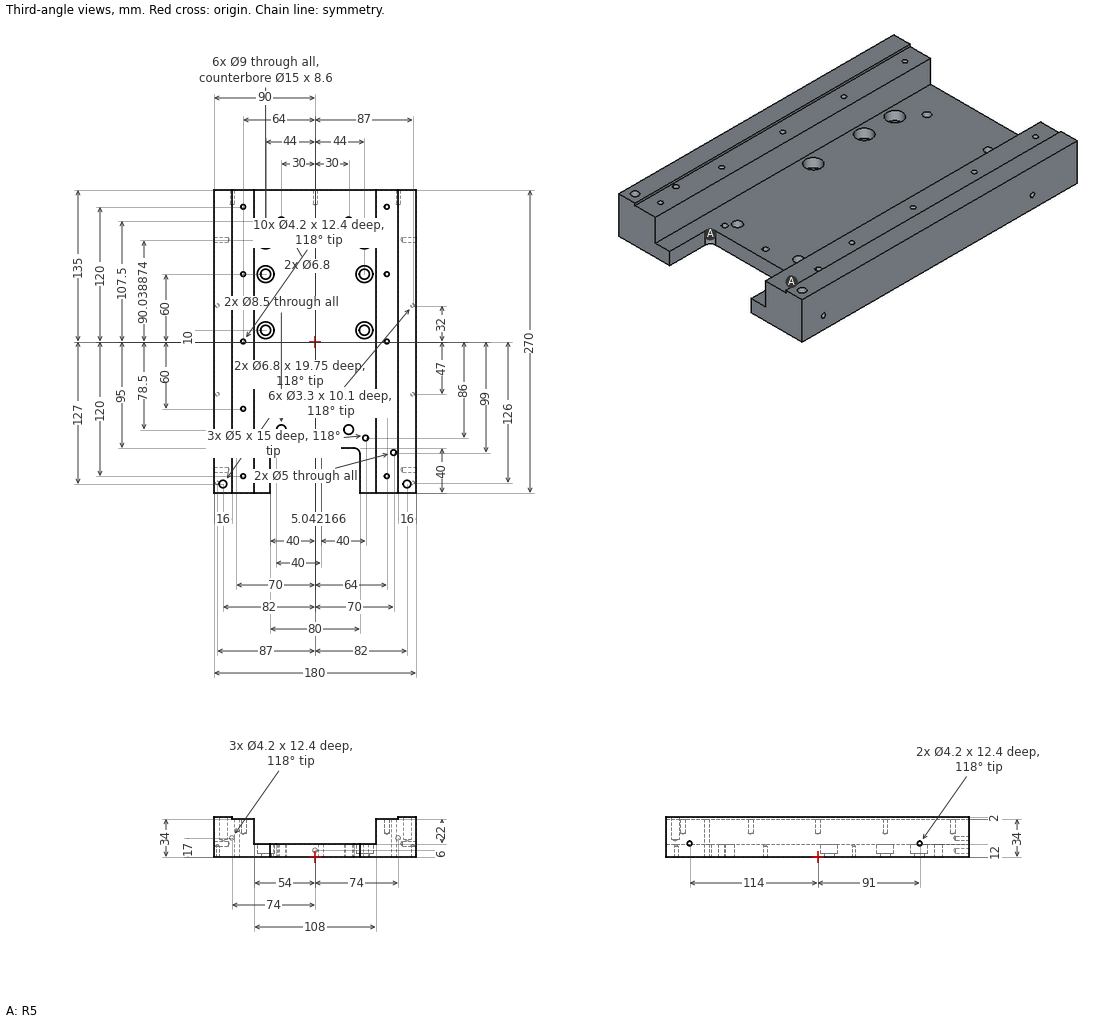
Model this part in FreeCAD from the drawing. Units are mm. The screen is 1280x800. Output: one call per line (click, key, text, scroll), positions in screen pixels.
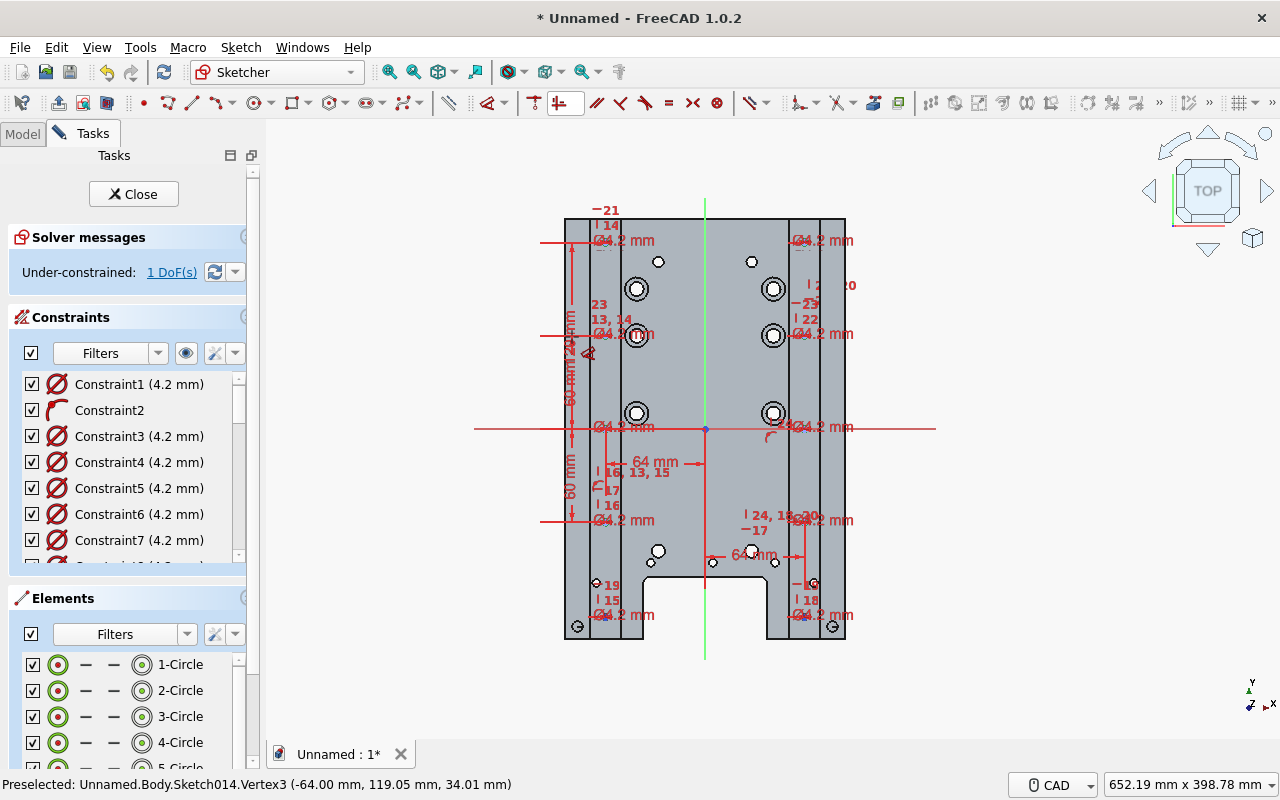
click(606, 617)
click(572, 523)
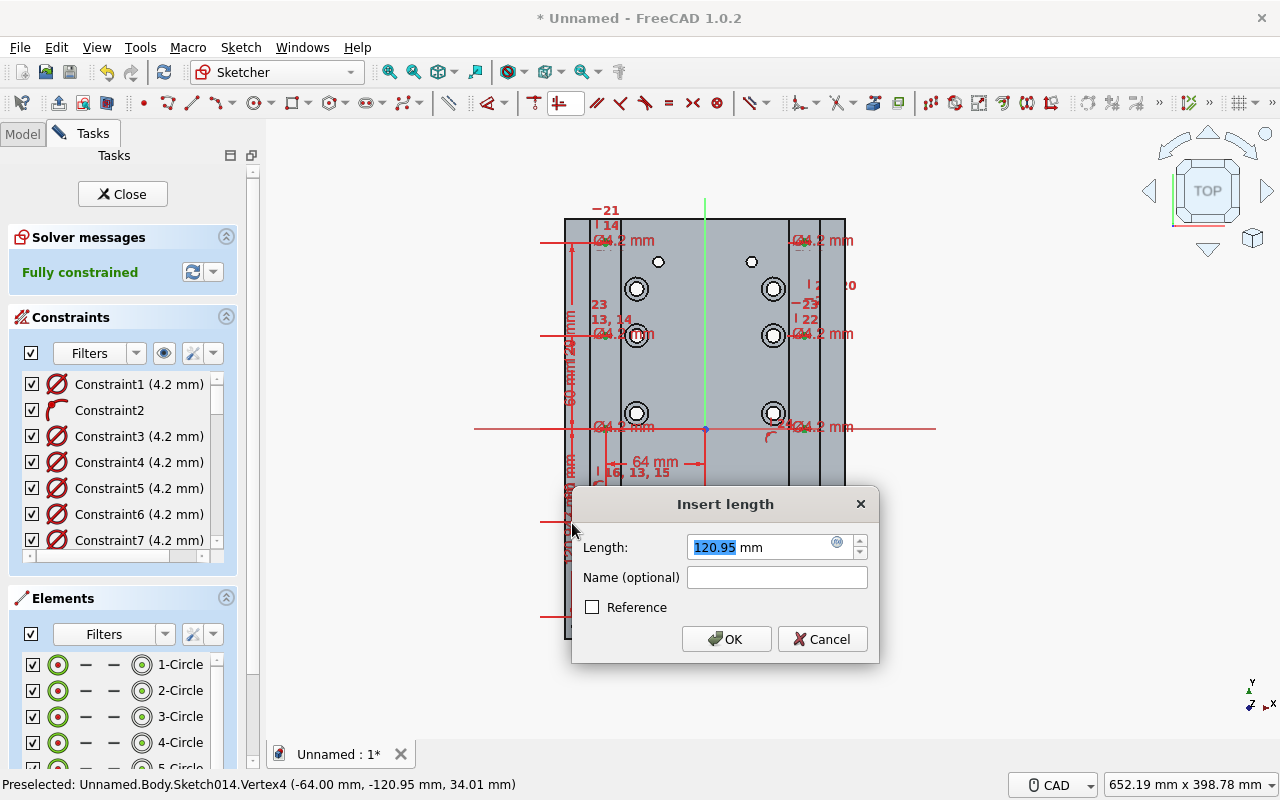
text(120)
key(Return)
key(Escape)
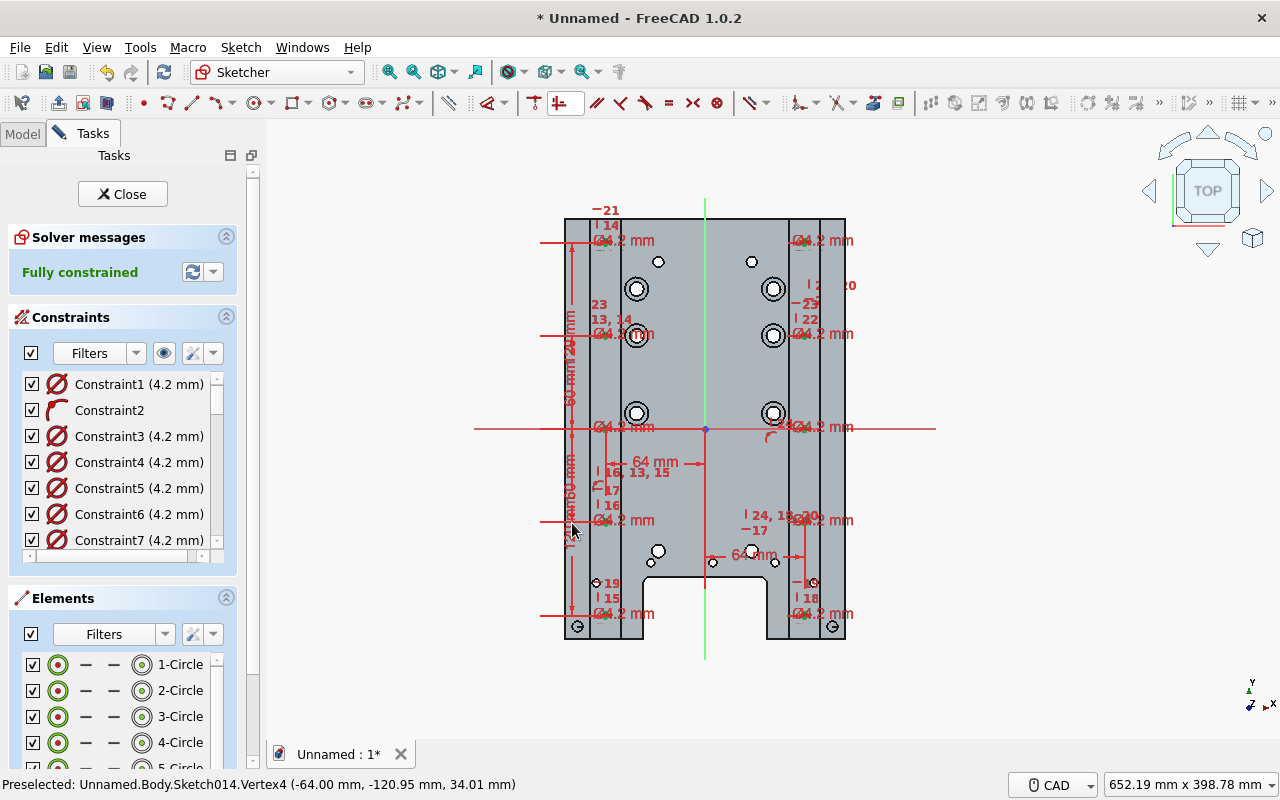
click(123, 194)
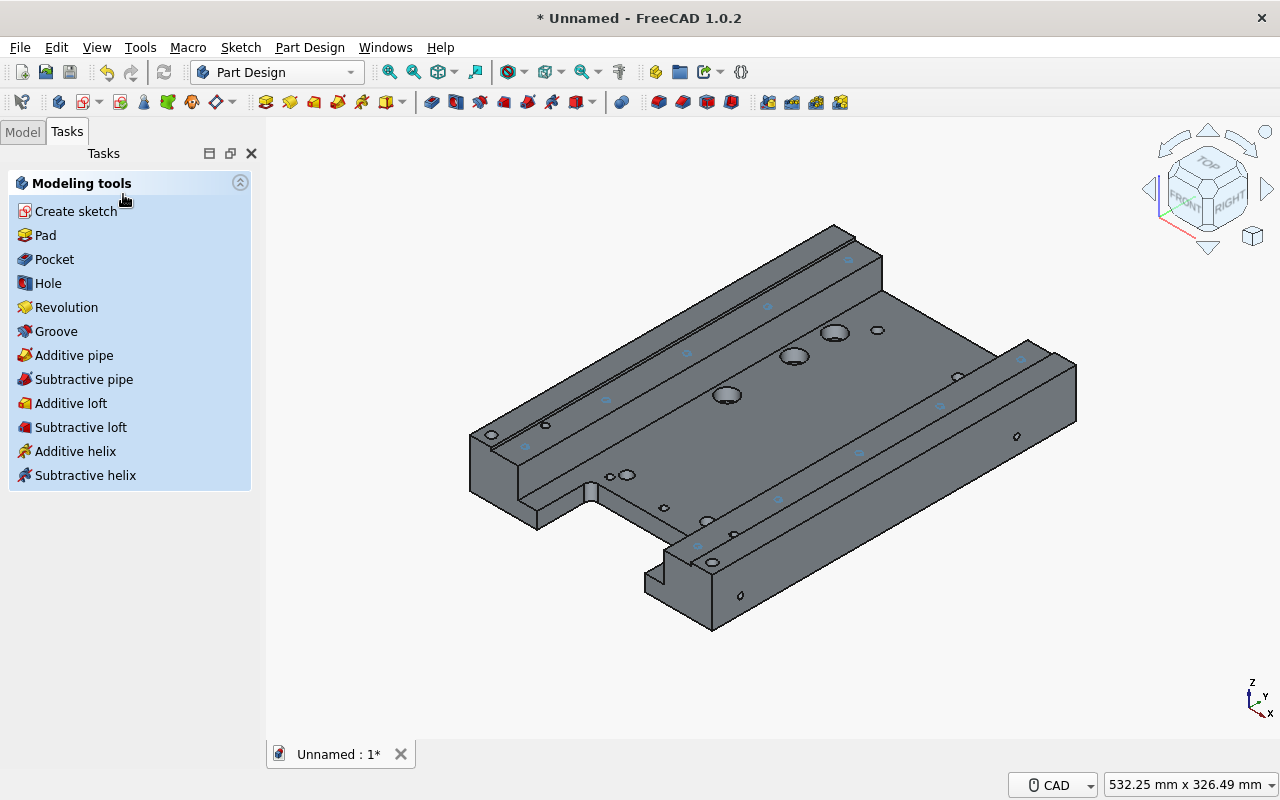
click(456, 102)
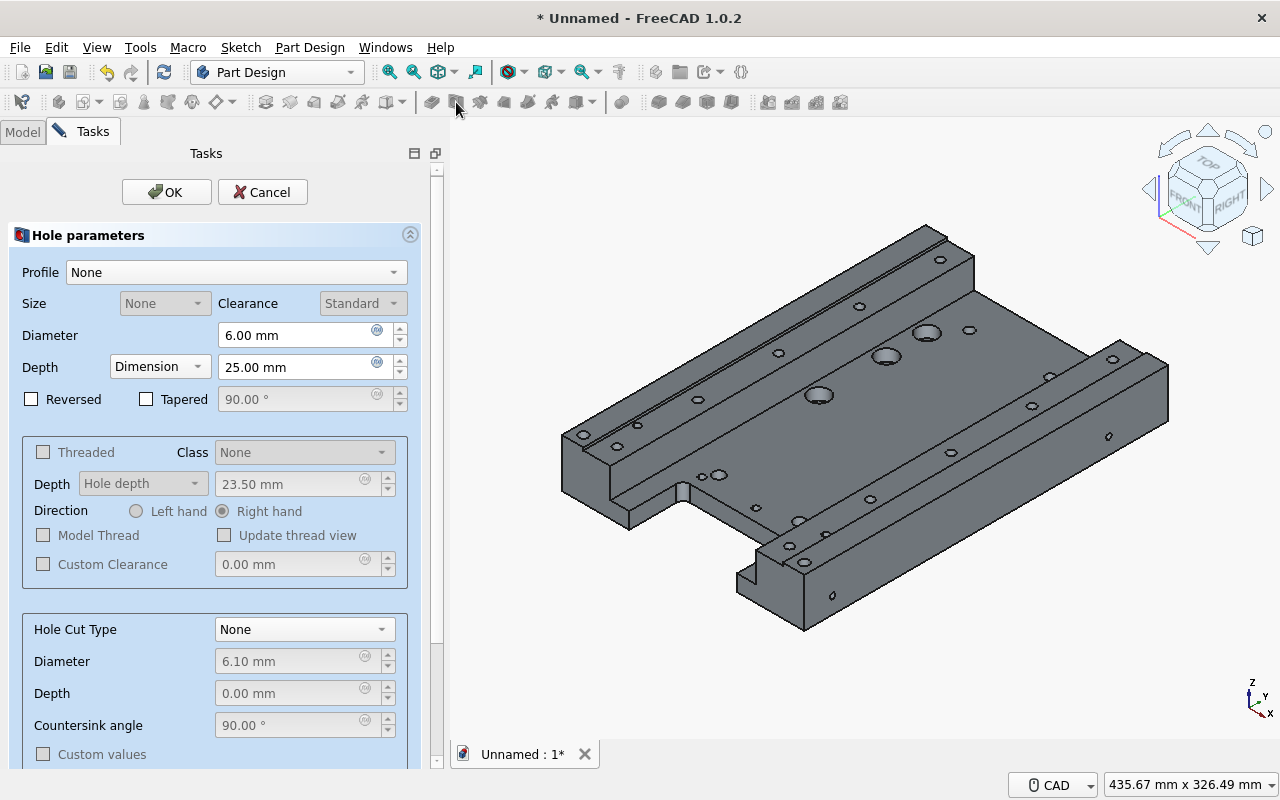
triple_click(305, 335)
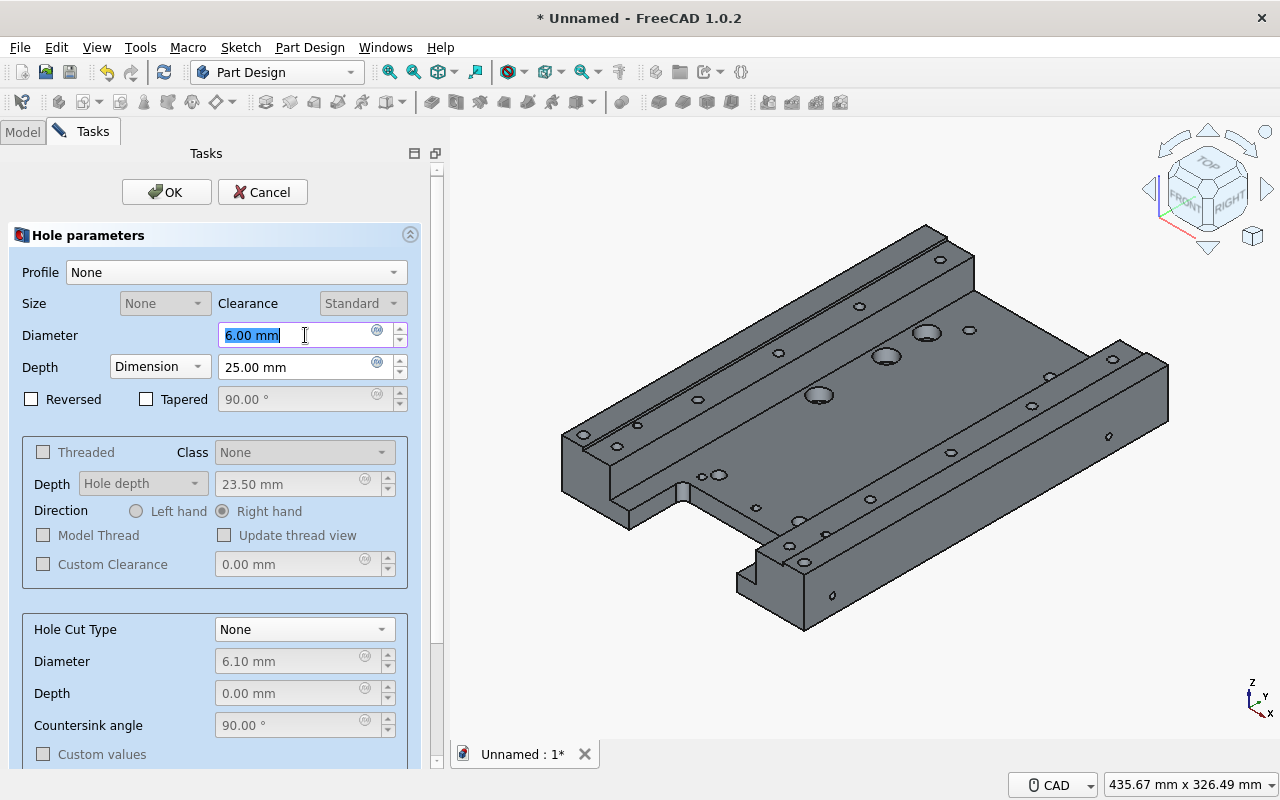
text(4.2)
key(Tab)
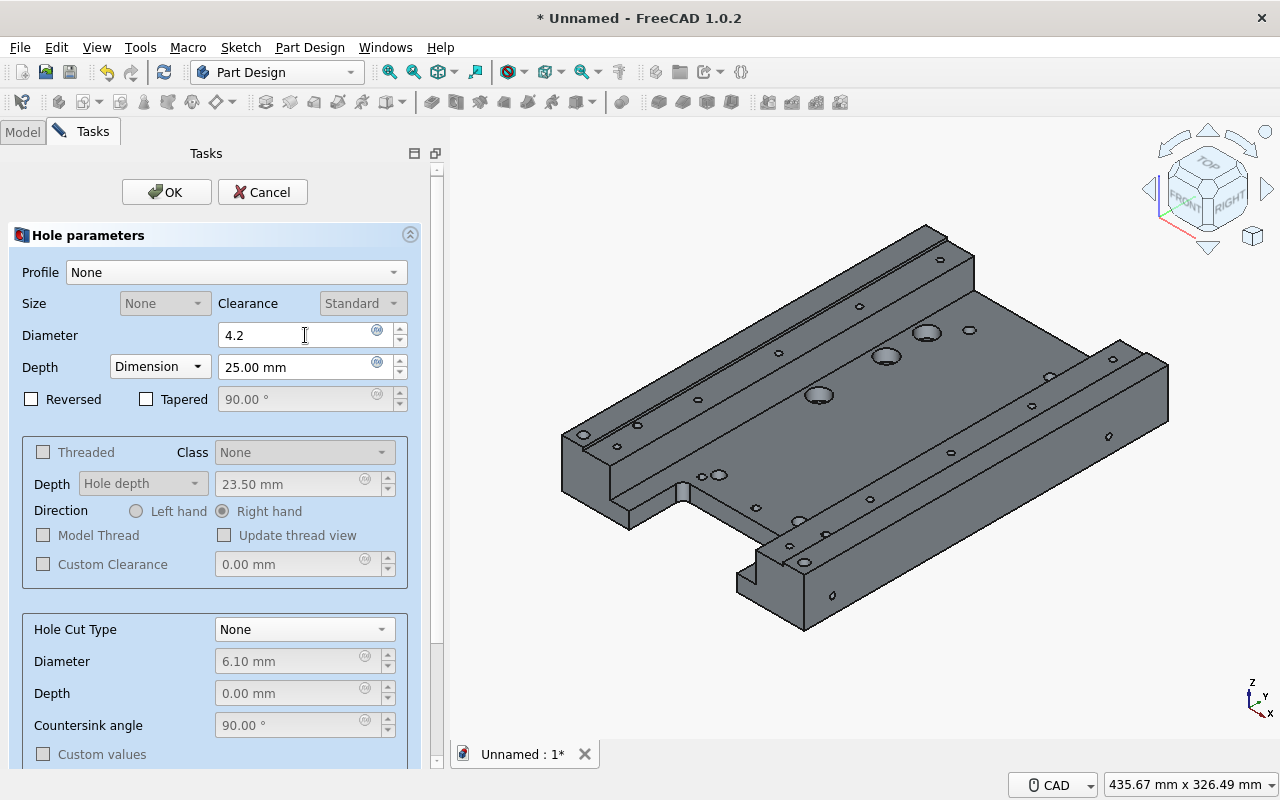
triple_click(305, 367)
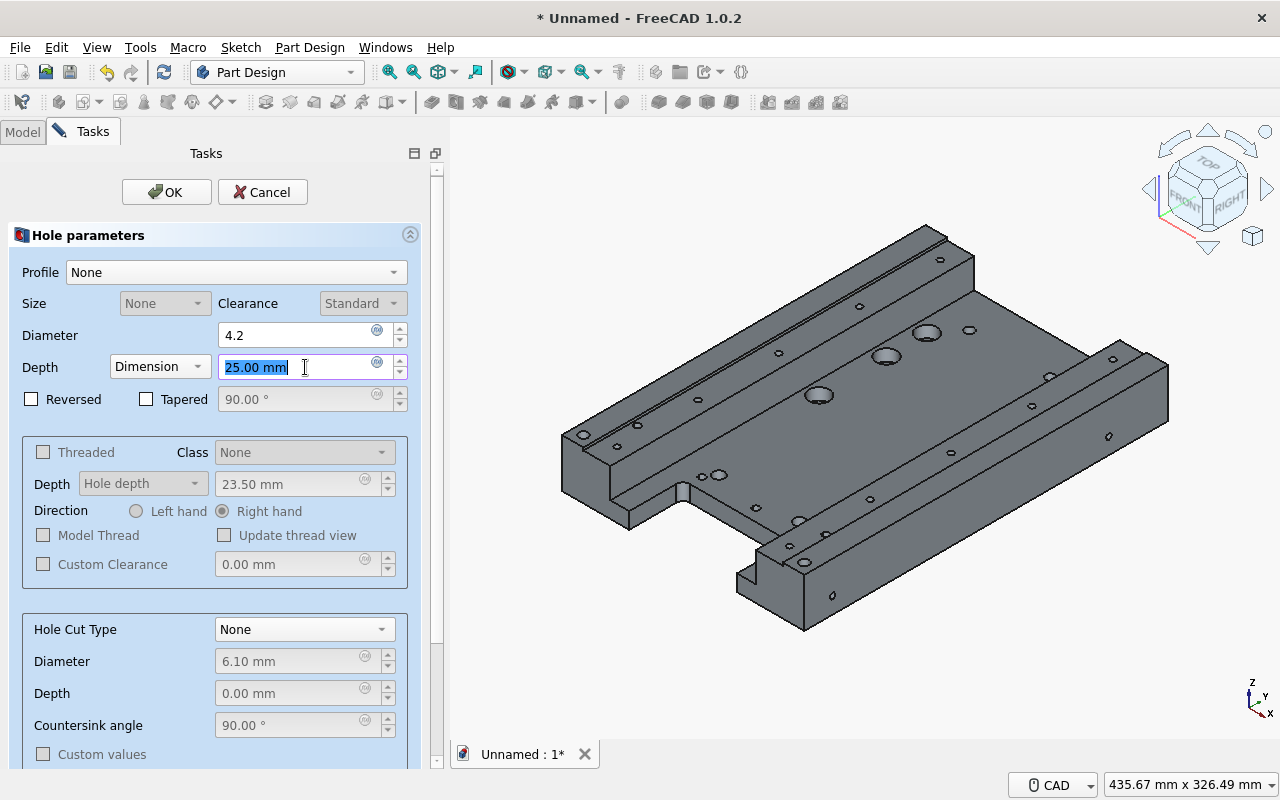
text(12.4)
key(Tab)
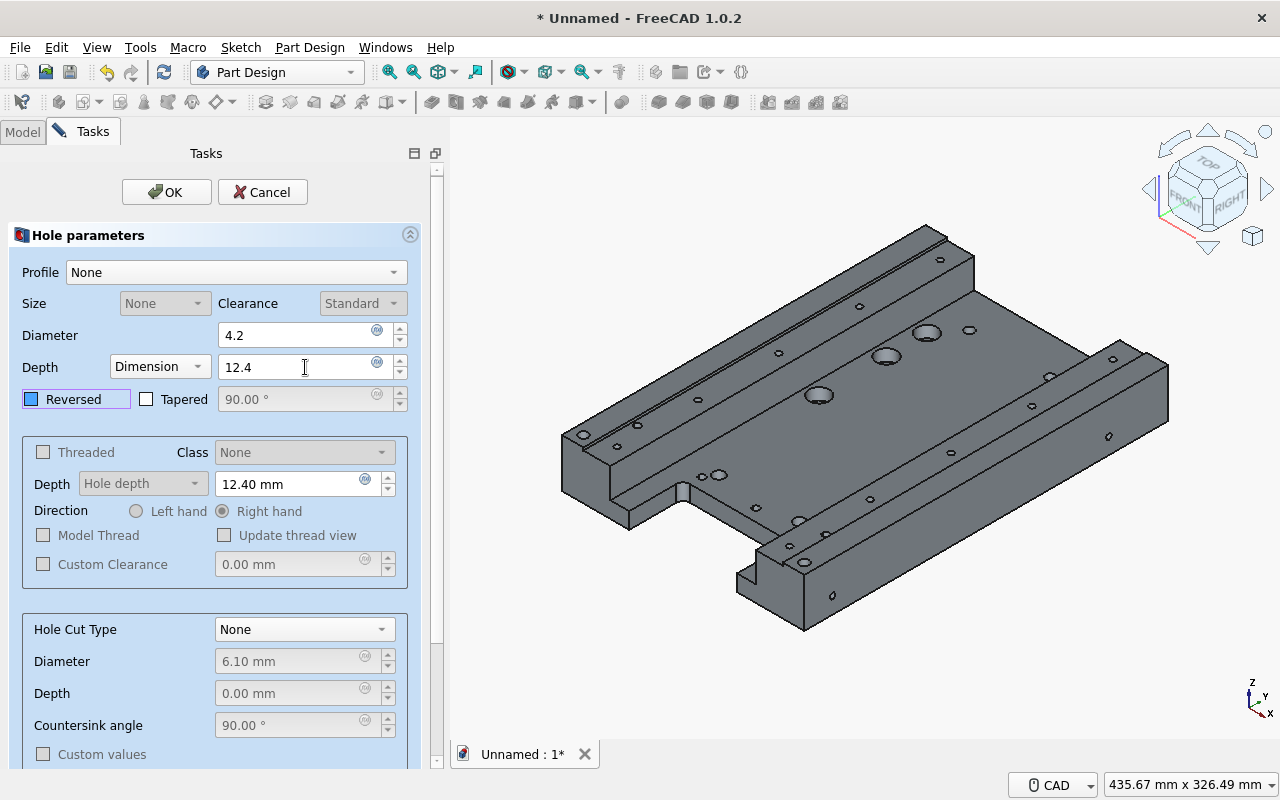
click(167, 192)